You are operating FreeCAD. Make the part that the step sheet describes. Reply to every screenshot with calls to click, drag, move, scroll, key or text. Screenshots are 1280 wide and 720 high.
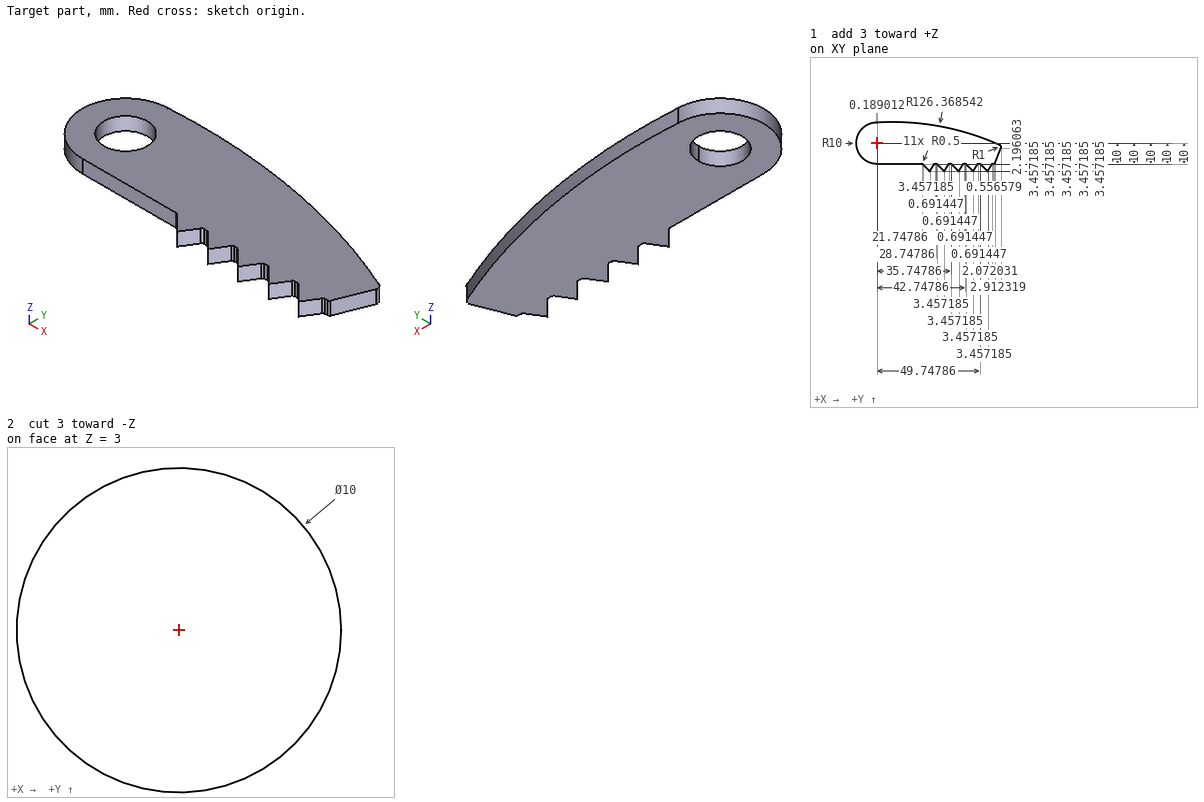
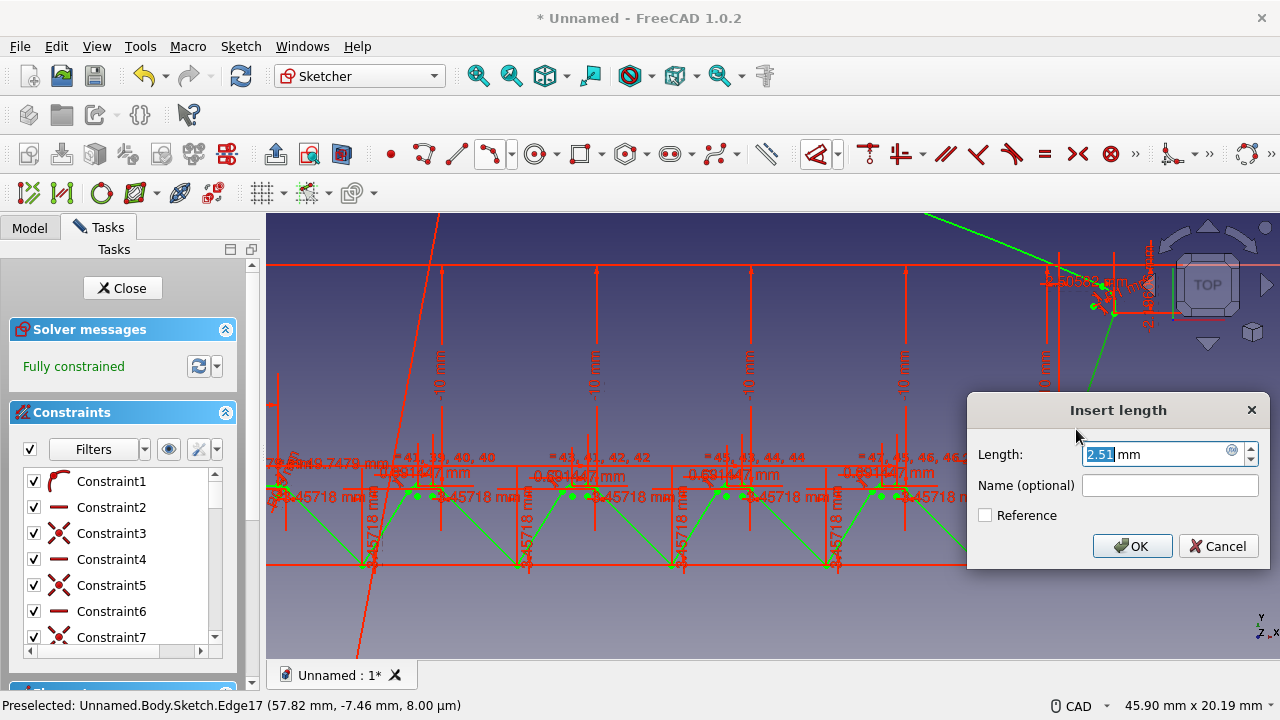
text(2.912319)
key(Return)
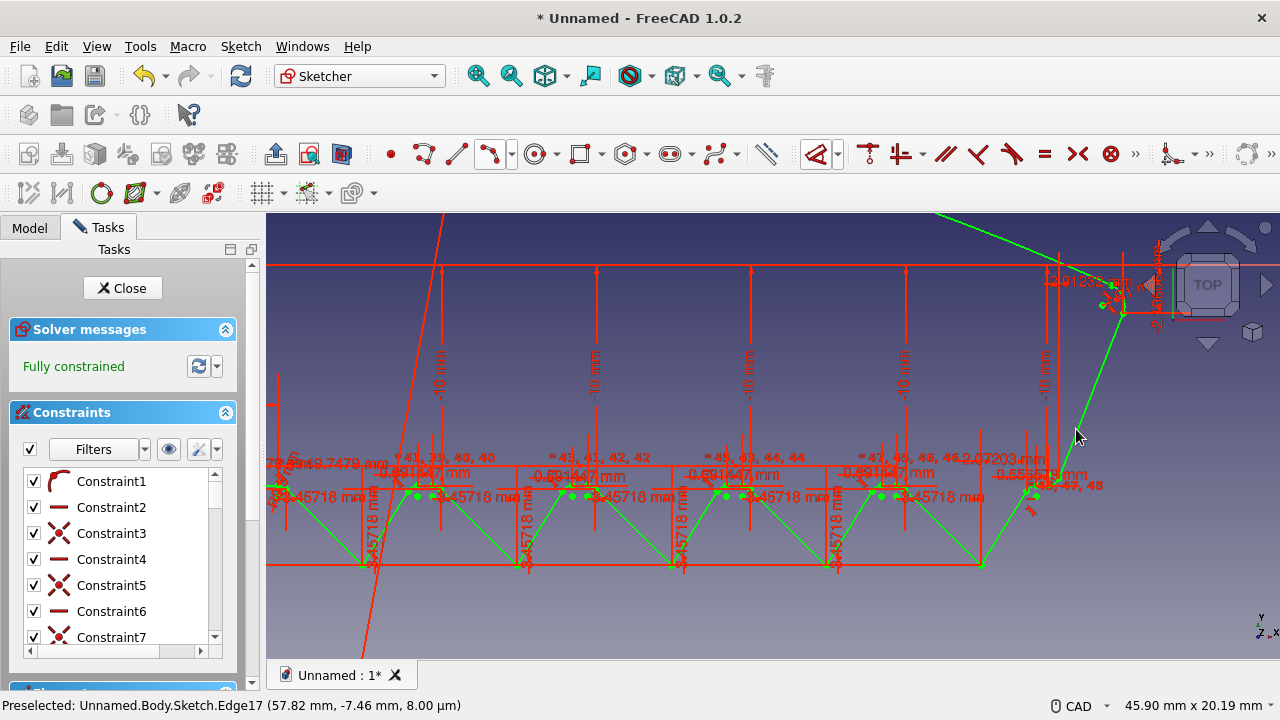
click(123, 288)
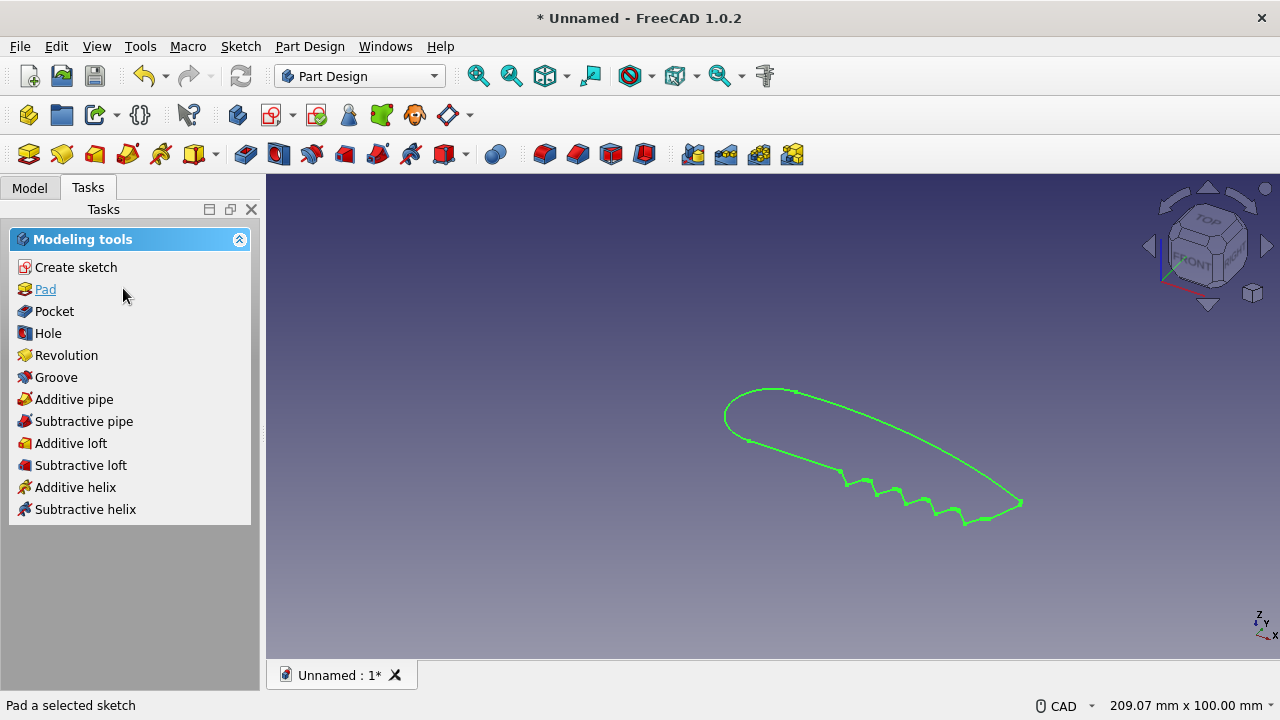
click(29, 154)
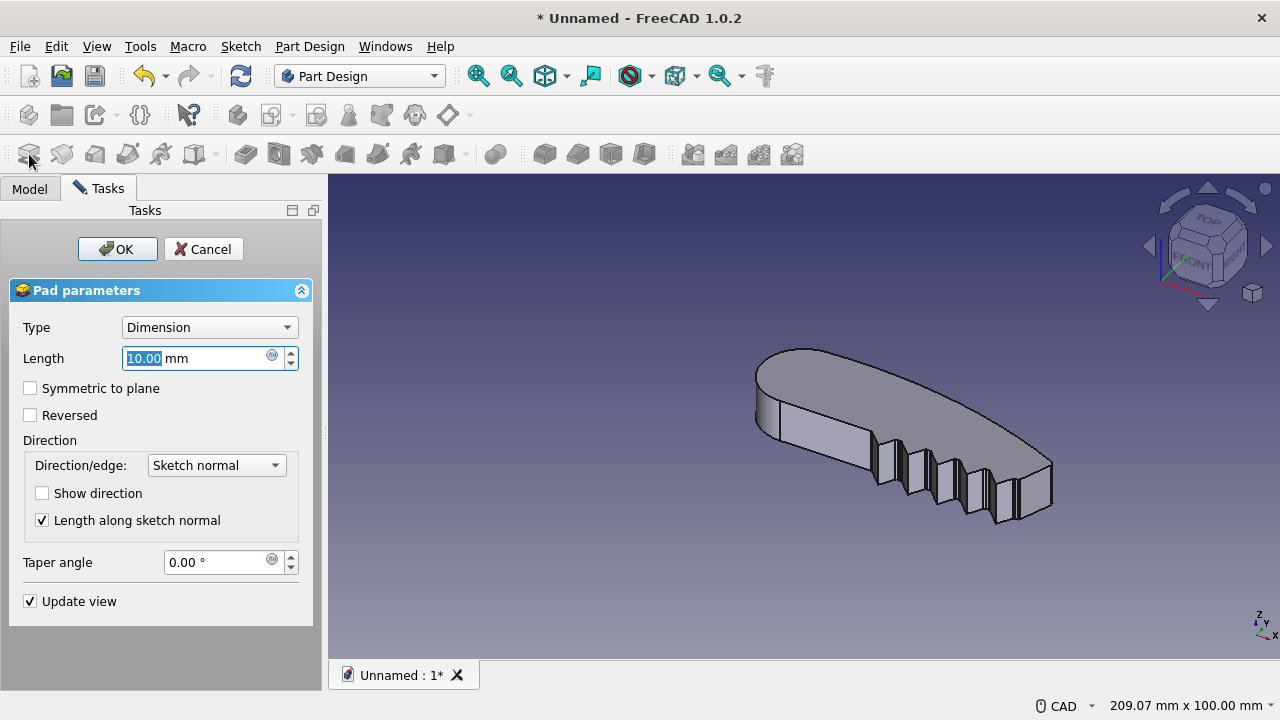
text(3)
key(Tab)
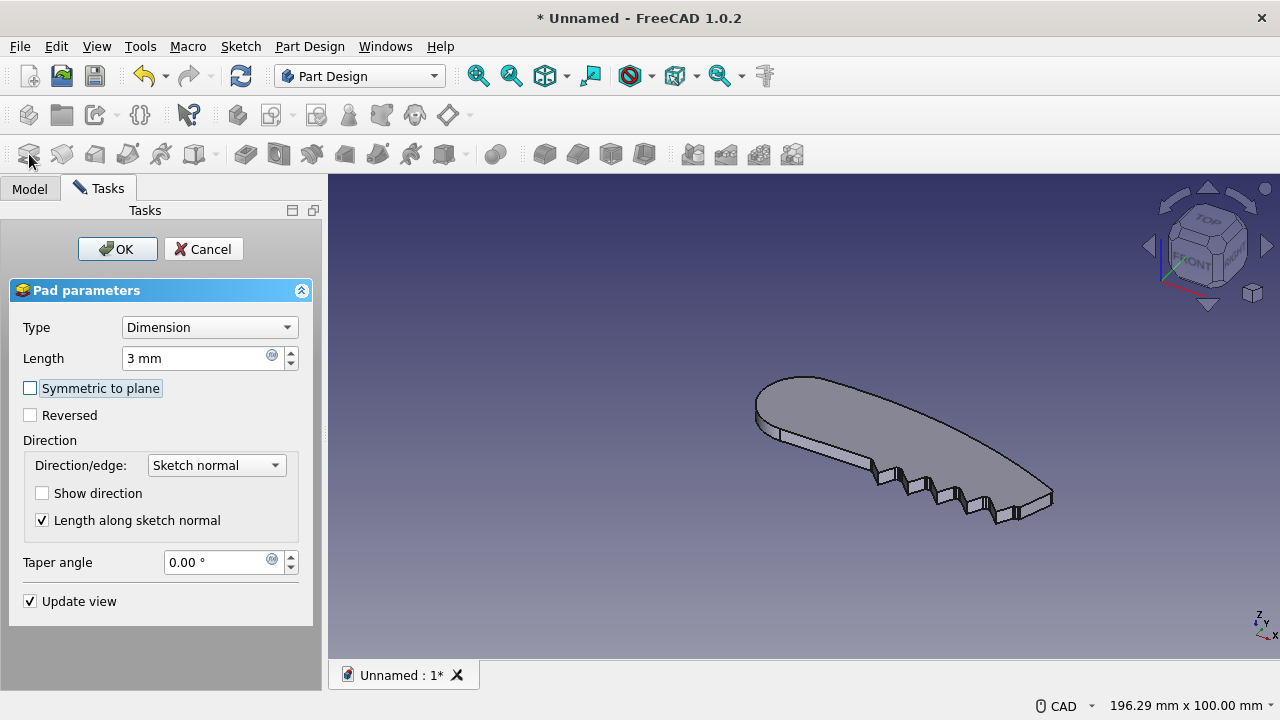
click(118, 249)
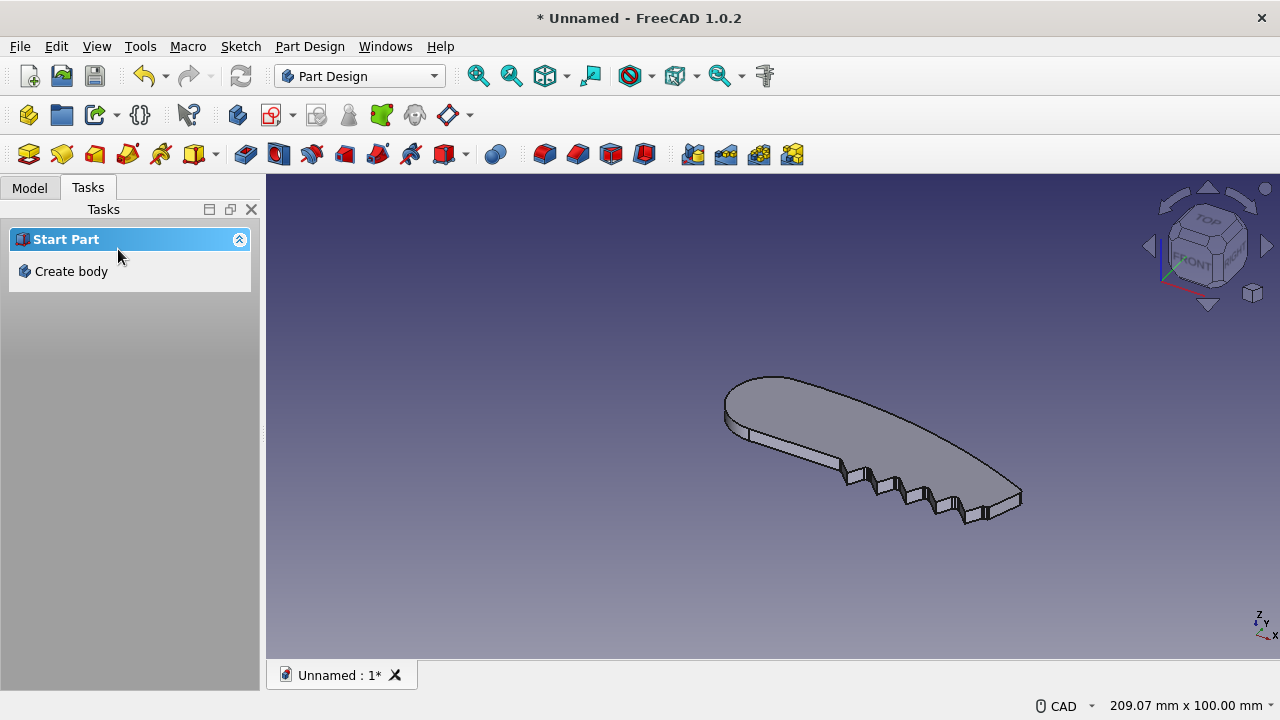
click(479, 76)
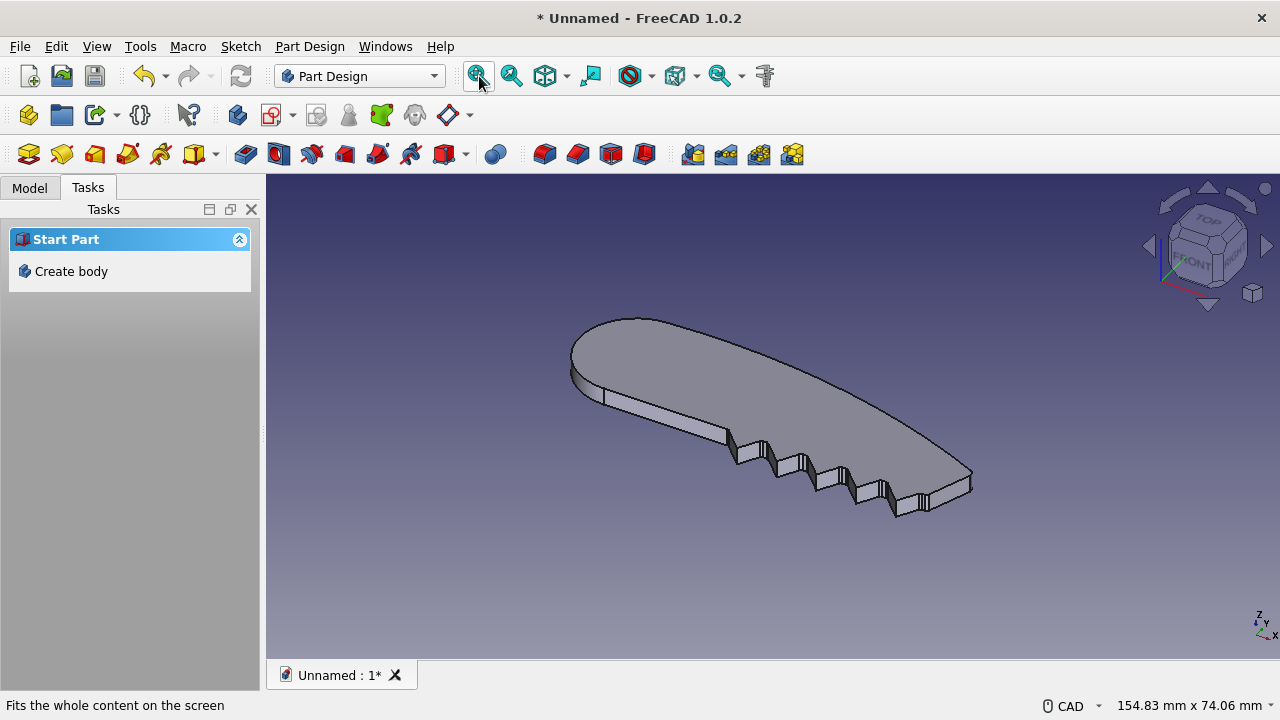
click(773, 407)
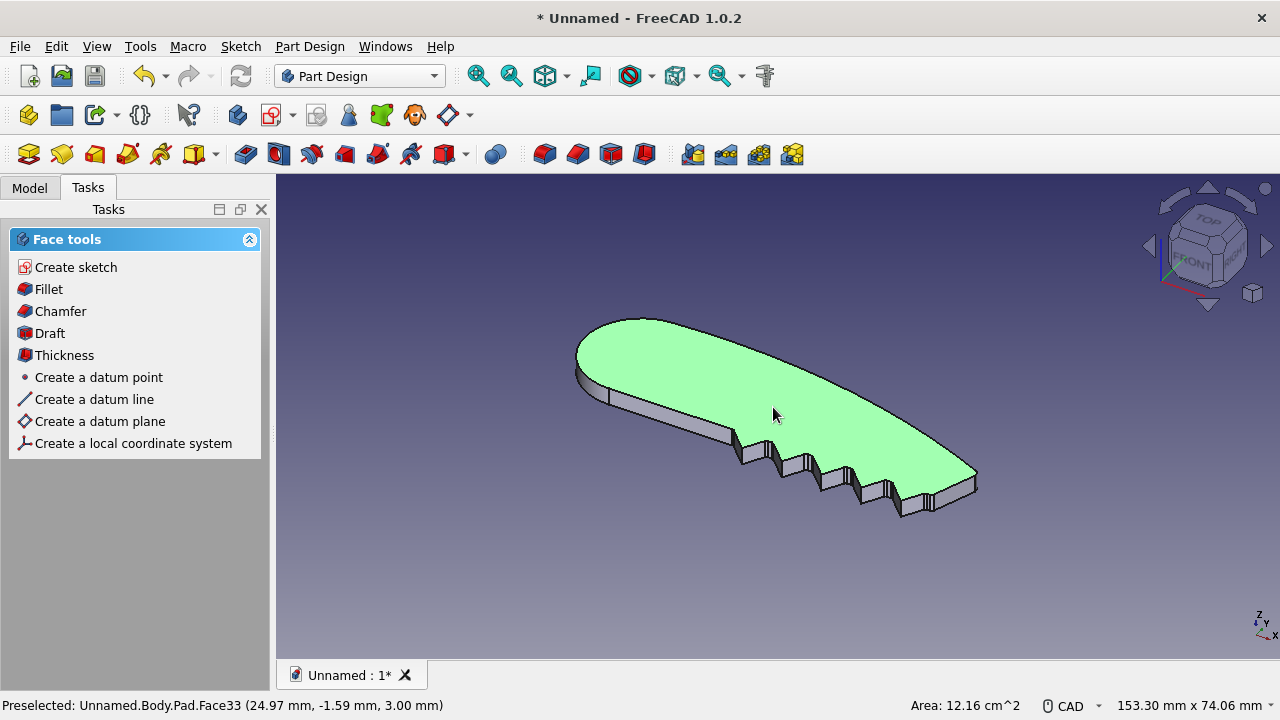
click(270, 116)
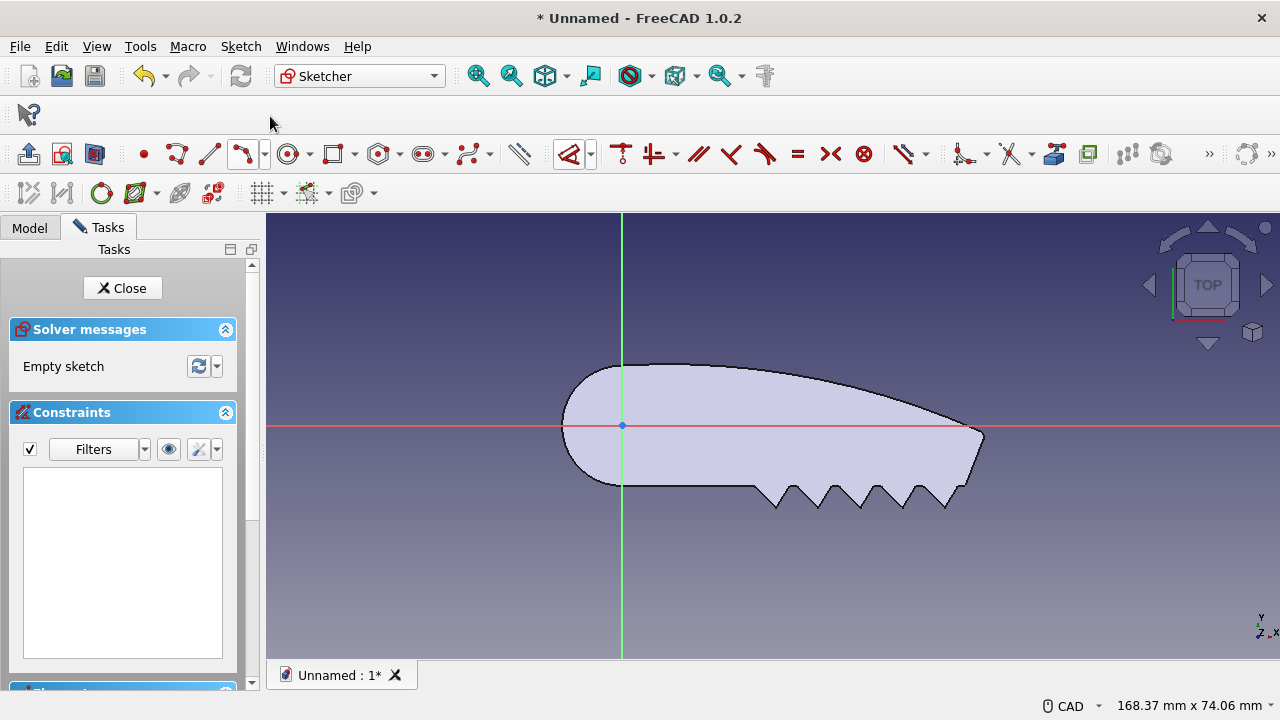
scroll(601, 423, up, 8)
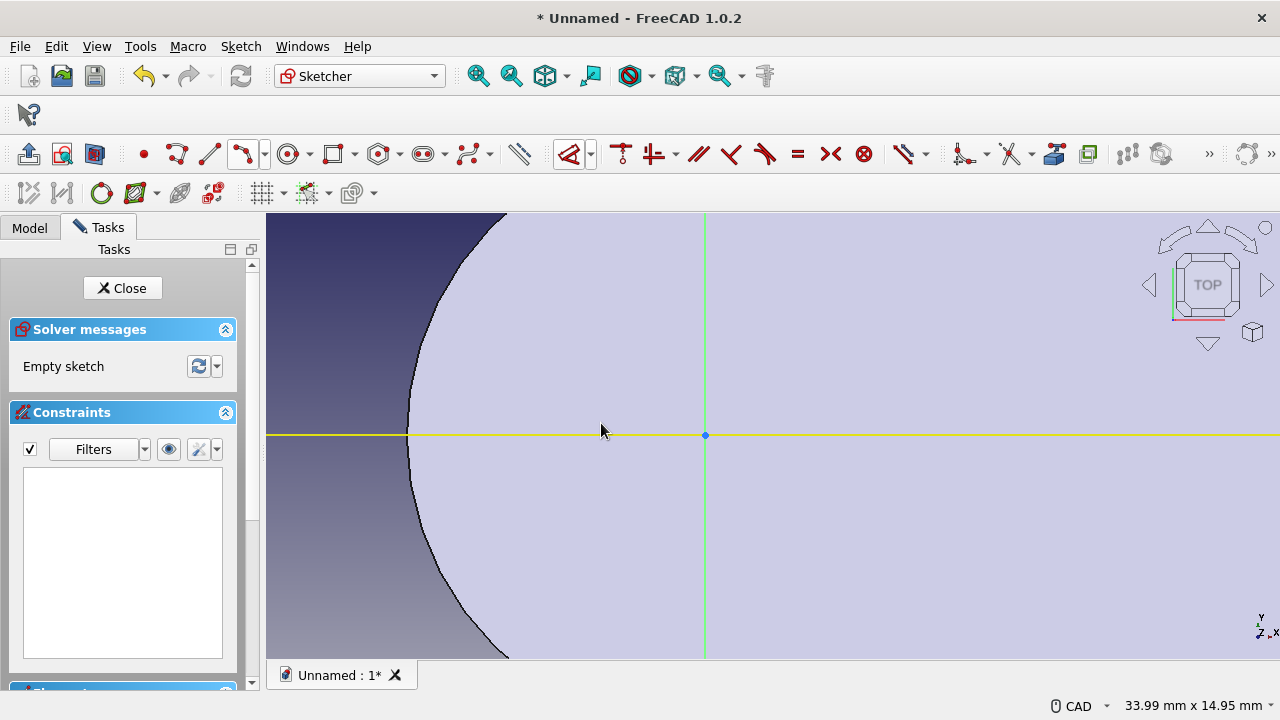
click(288, 154)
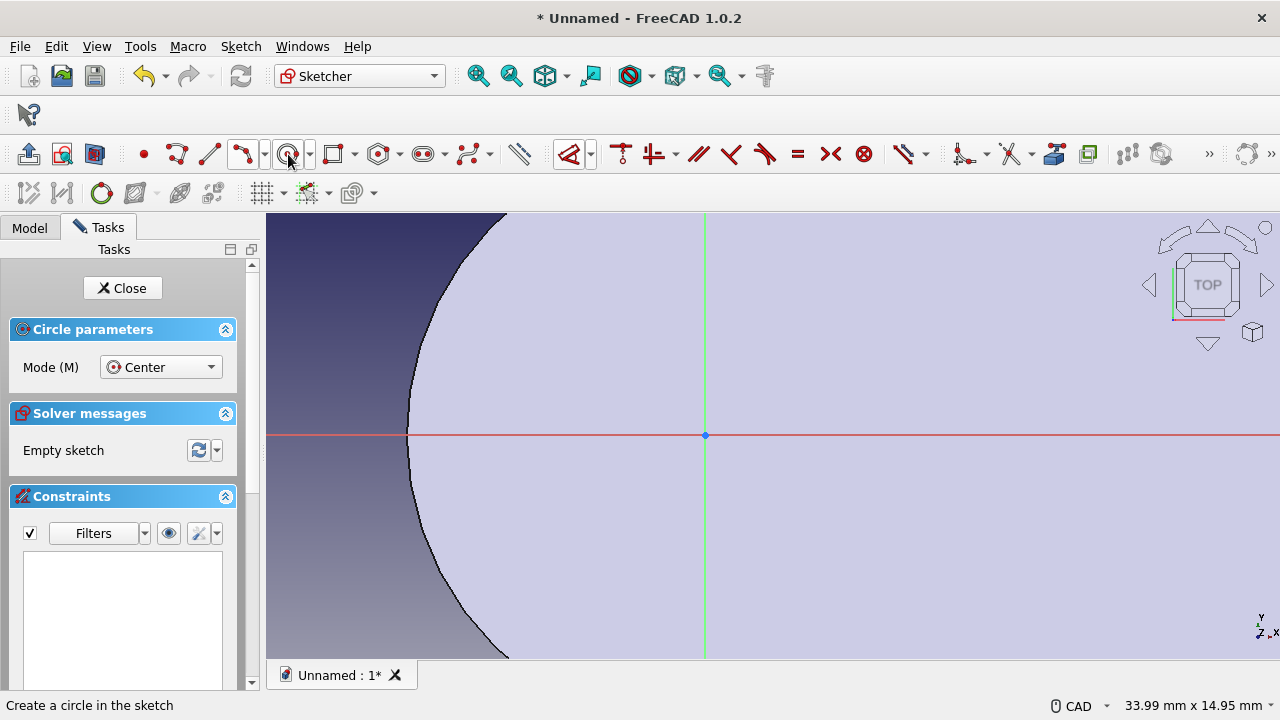
click(705, 435)
click(810, 330)
key(Escape)